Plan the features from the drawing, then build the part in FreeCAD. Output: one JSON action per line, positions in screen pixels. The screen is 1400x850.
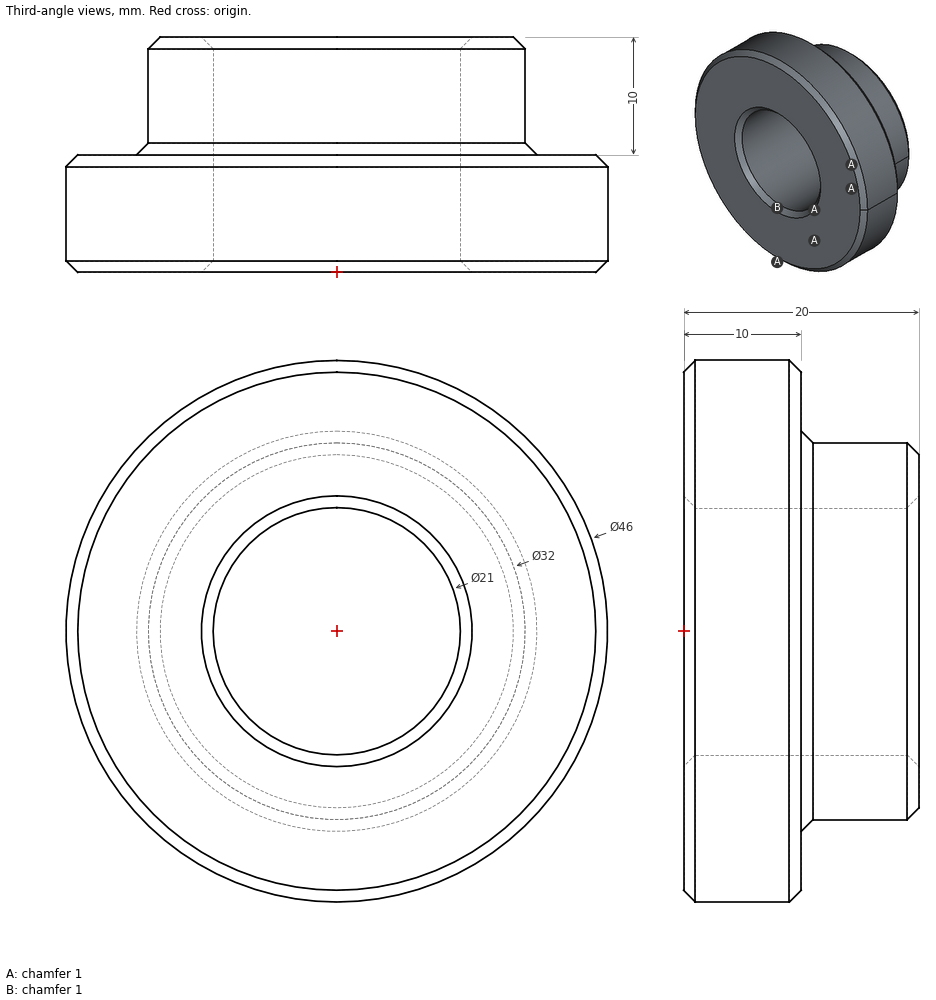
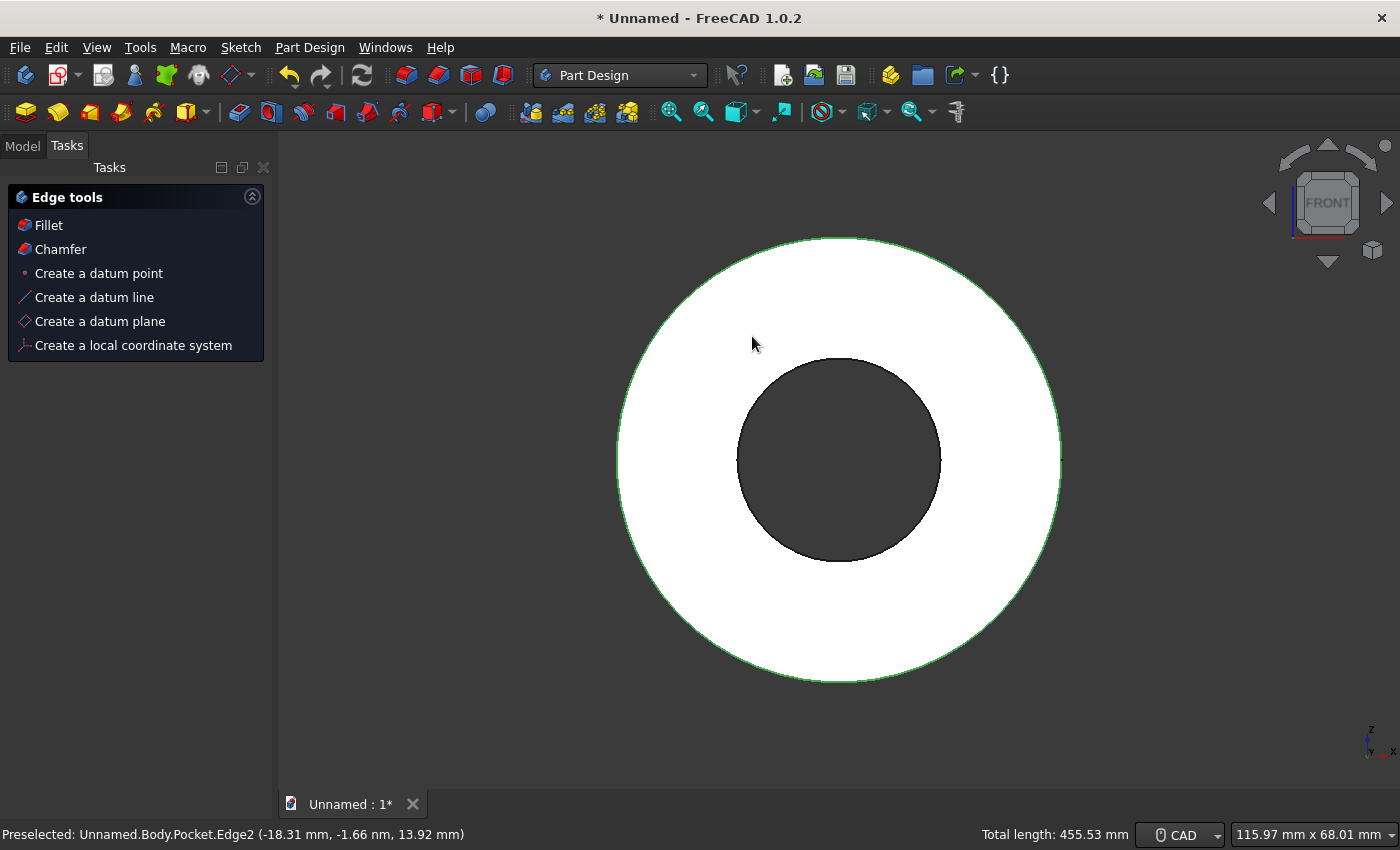
{"action": "key", "text": "3"}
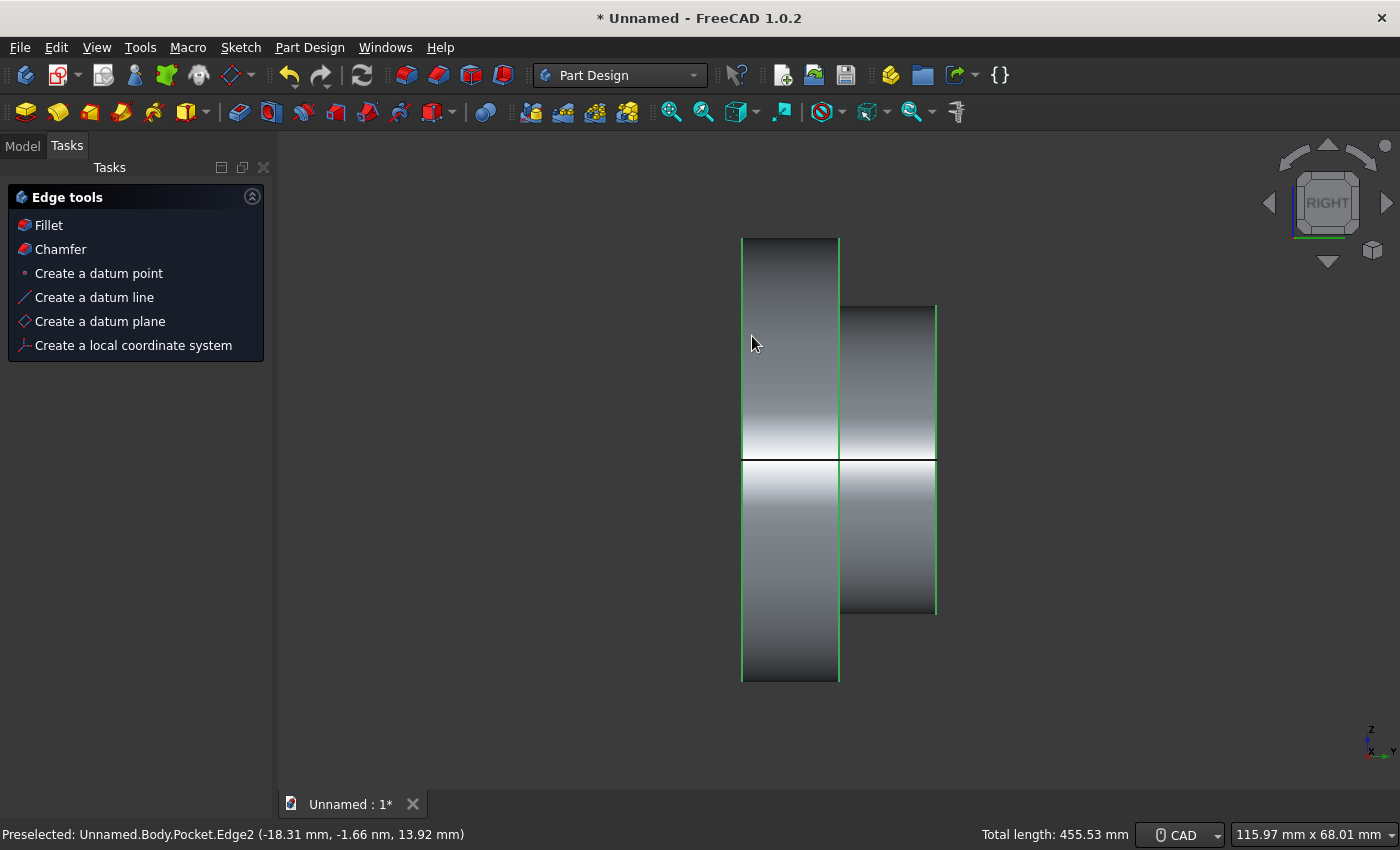
{"action": "key", "text": "5"}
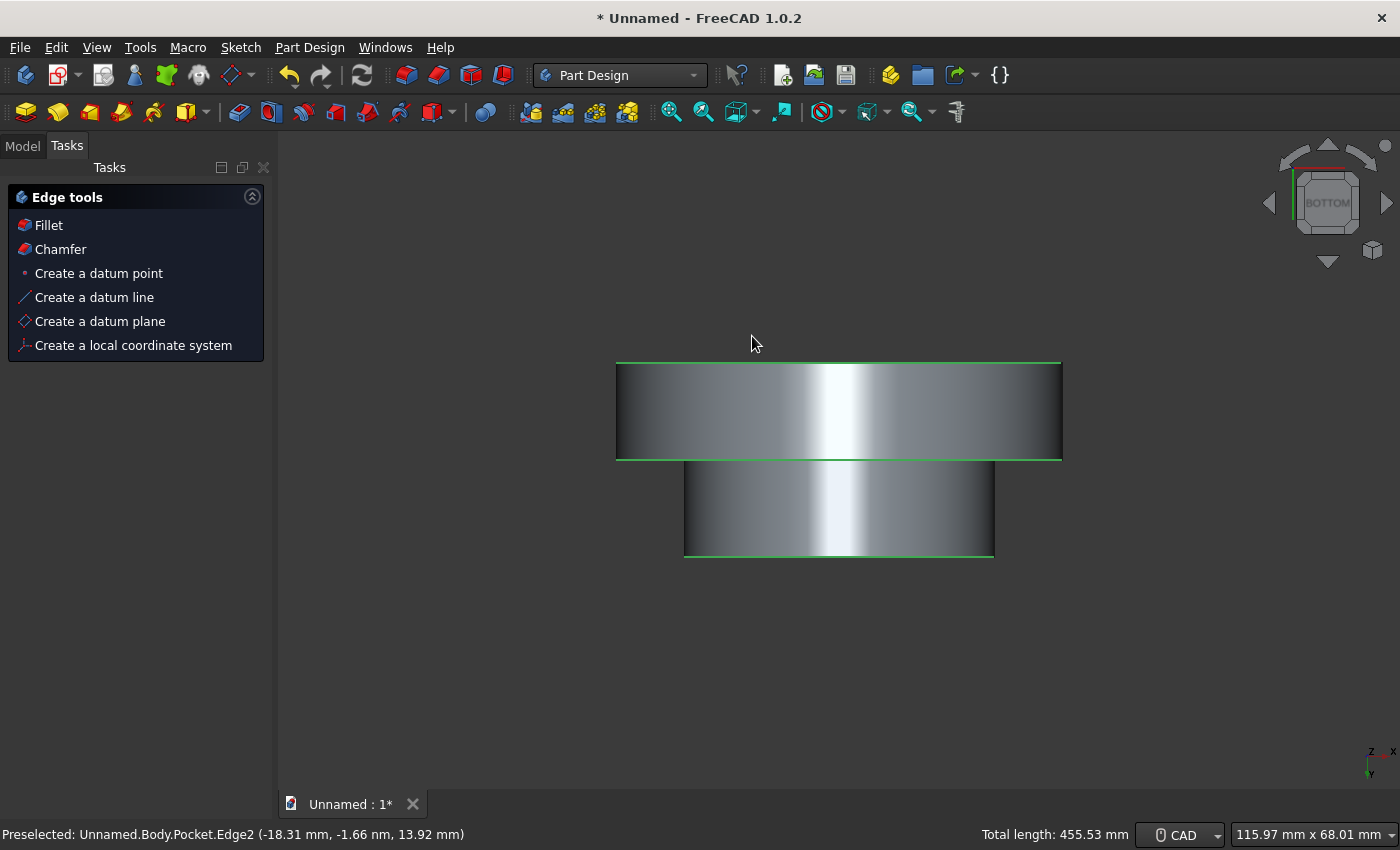
{"action": "left_click", "coordinate": [672, 112]}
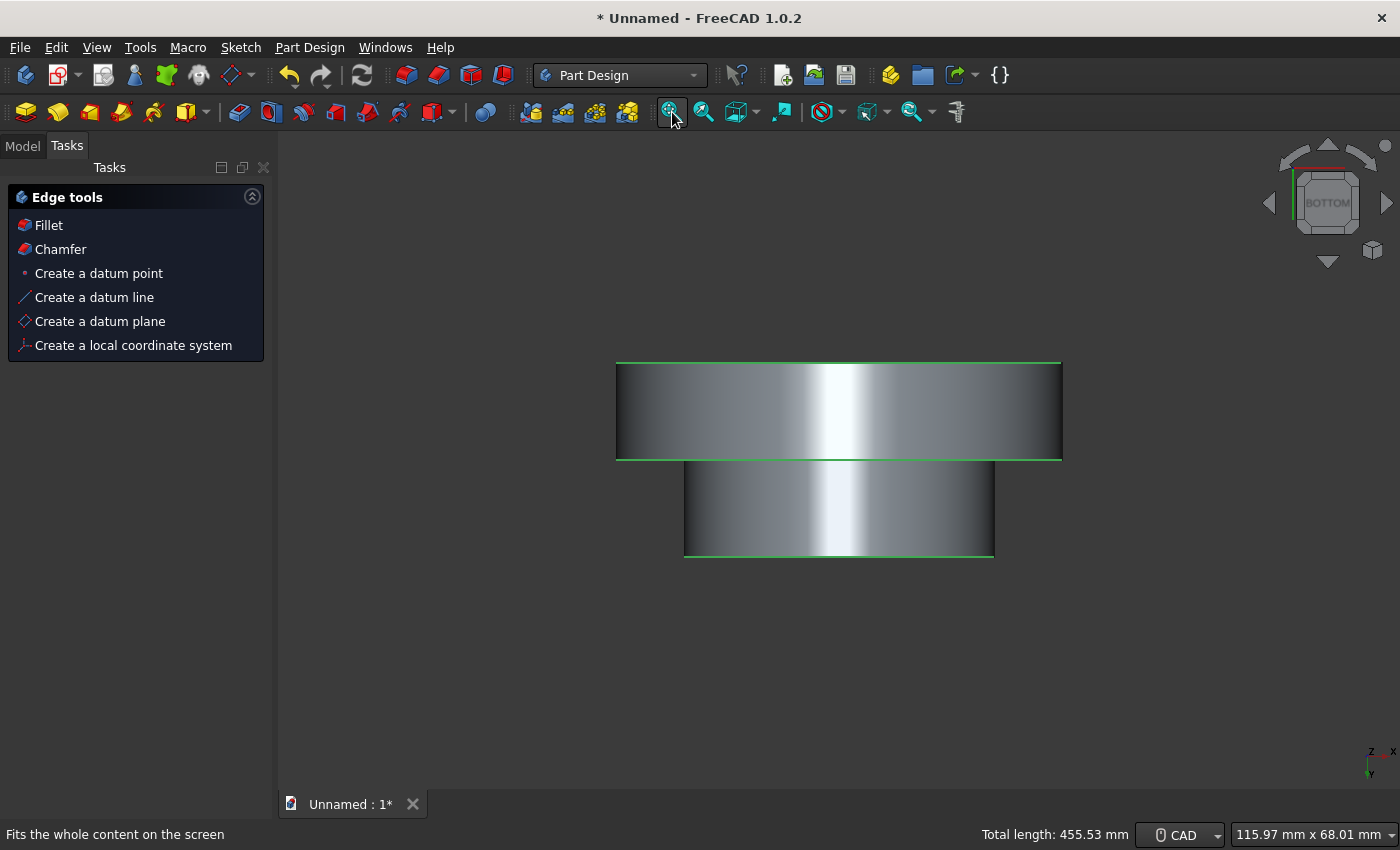
{"action": "key", "text": "4"}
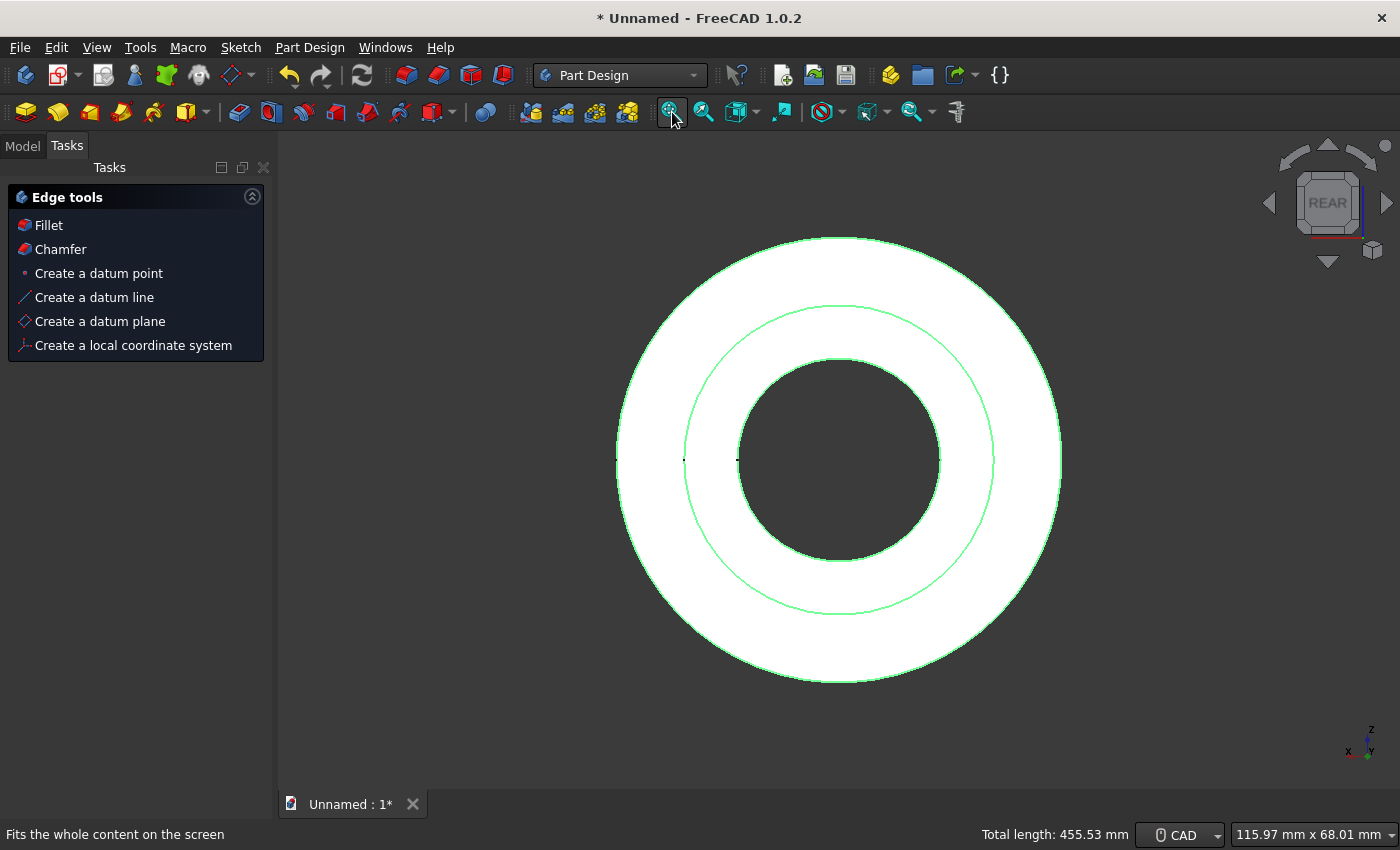
{"action": "key", "text": "6"}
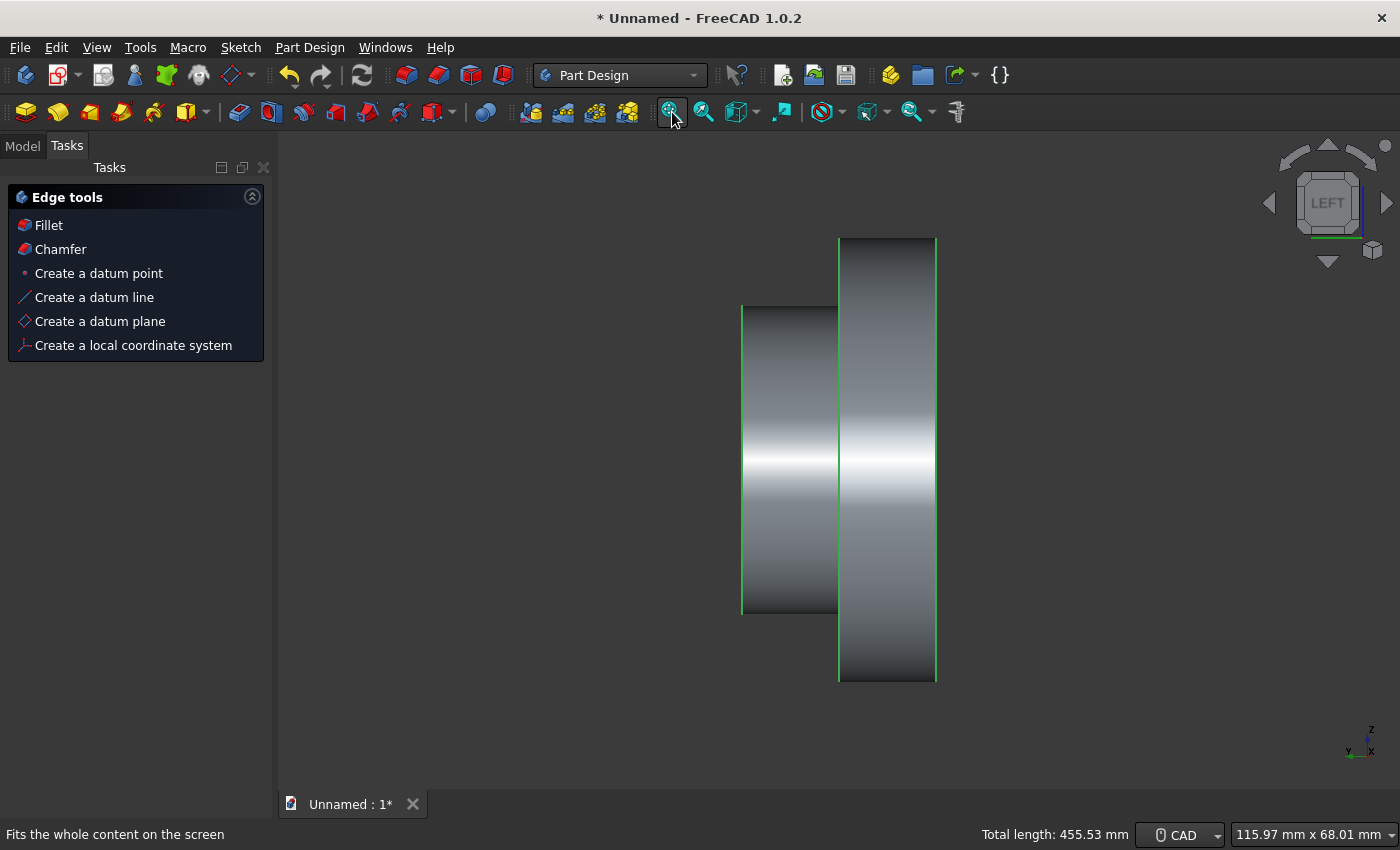
{"action": "key", "text": "v 3"}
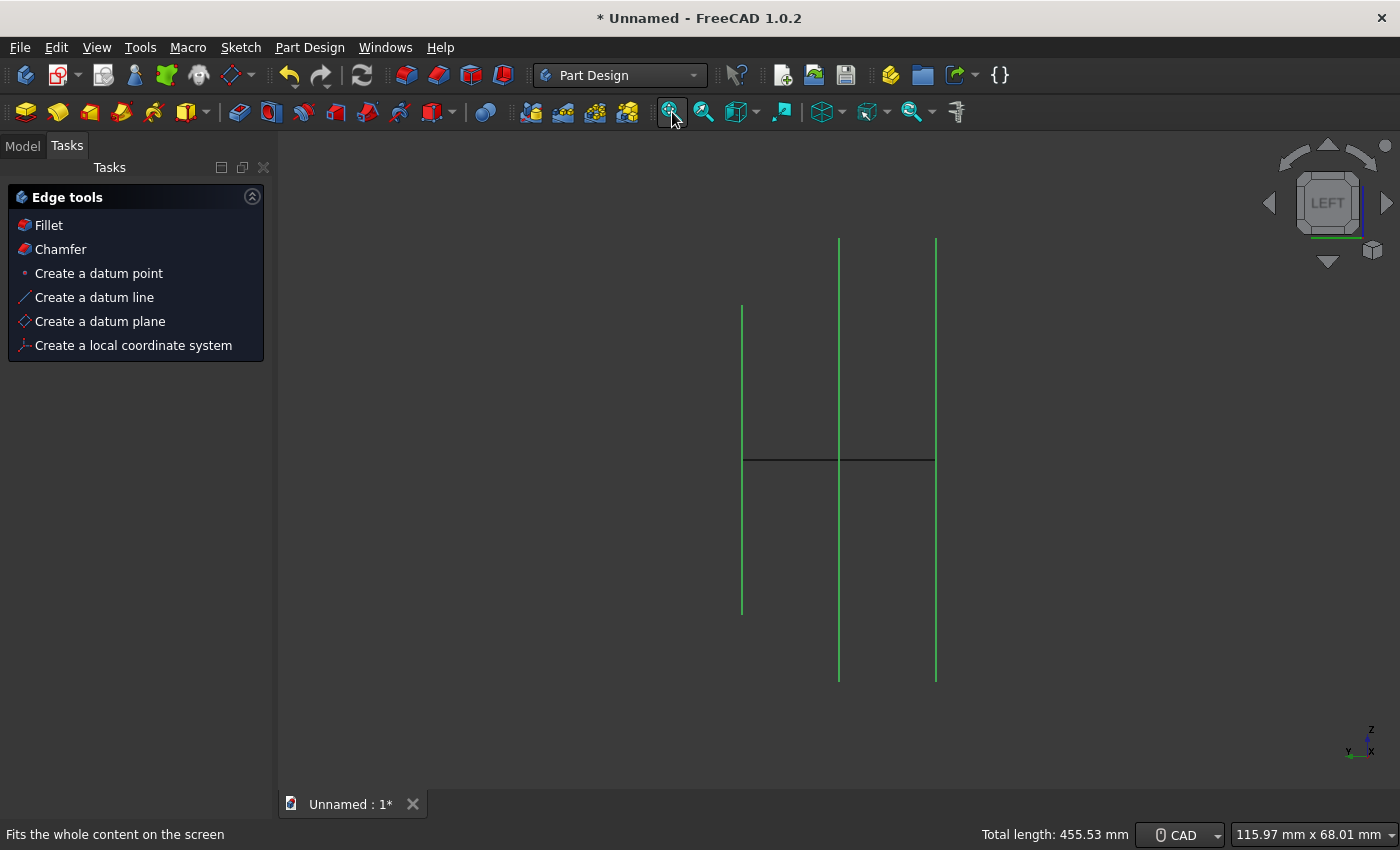
{"action": "key", "text": "0"}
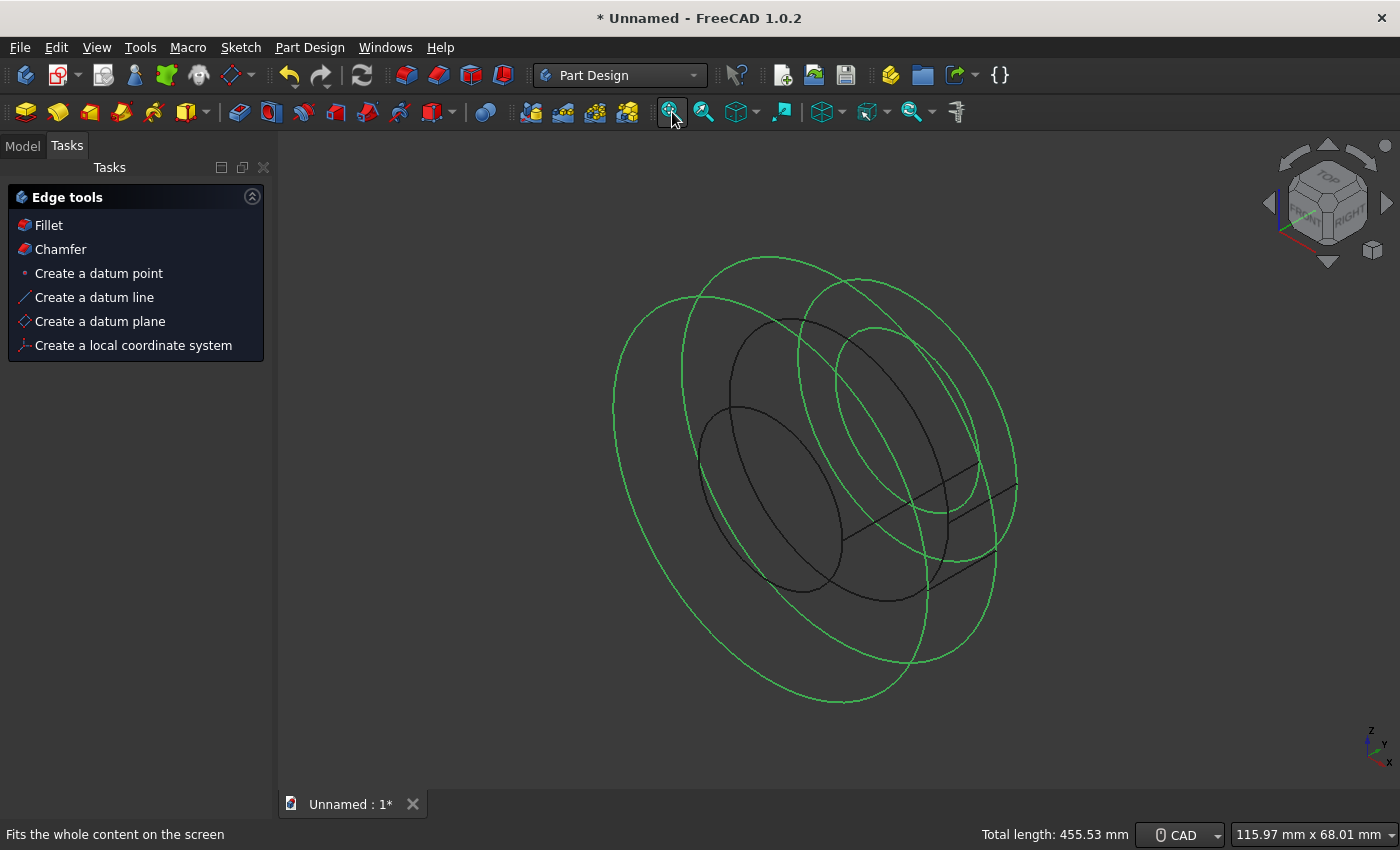
{"action": "left_click", "coordinate": [730, 396], "text": "ctrl"}